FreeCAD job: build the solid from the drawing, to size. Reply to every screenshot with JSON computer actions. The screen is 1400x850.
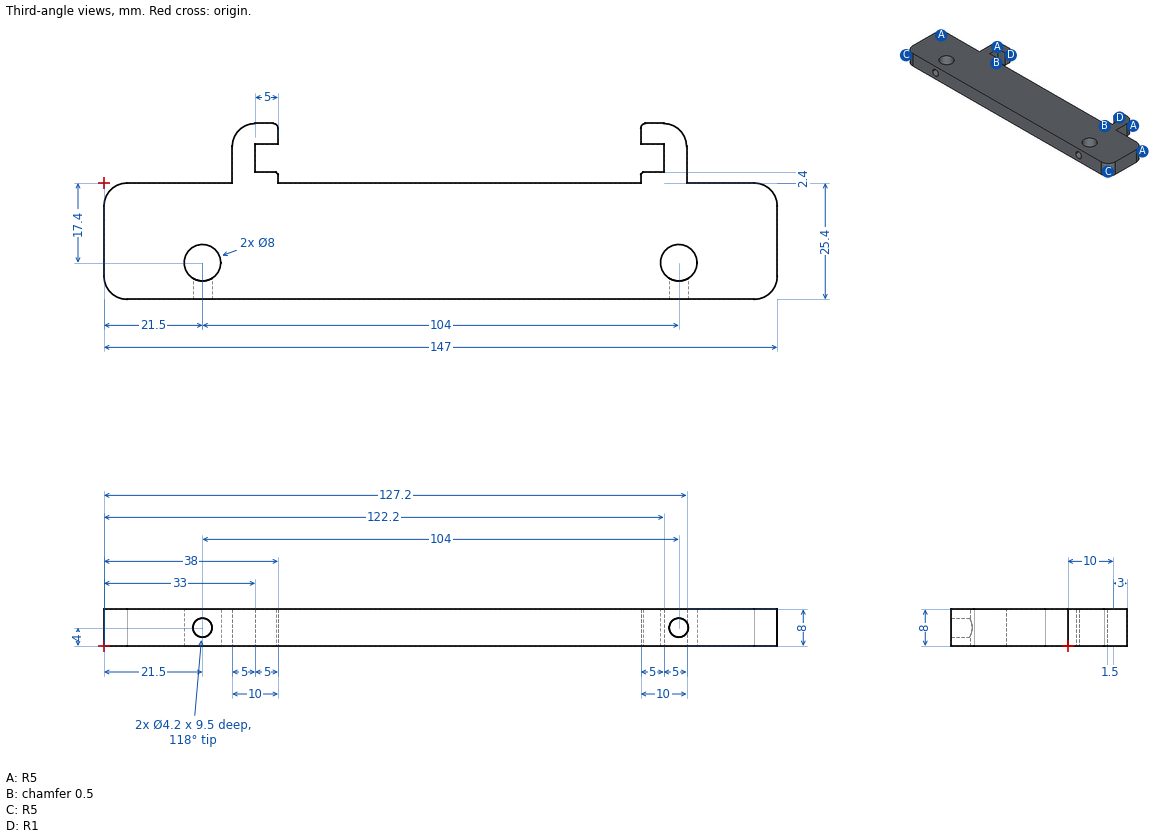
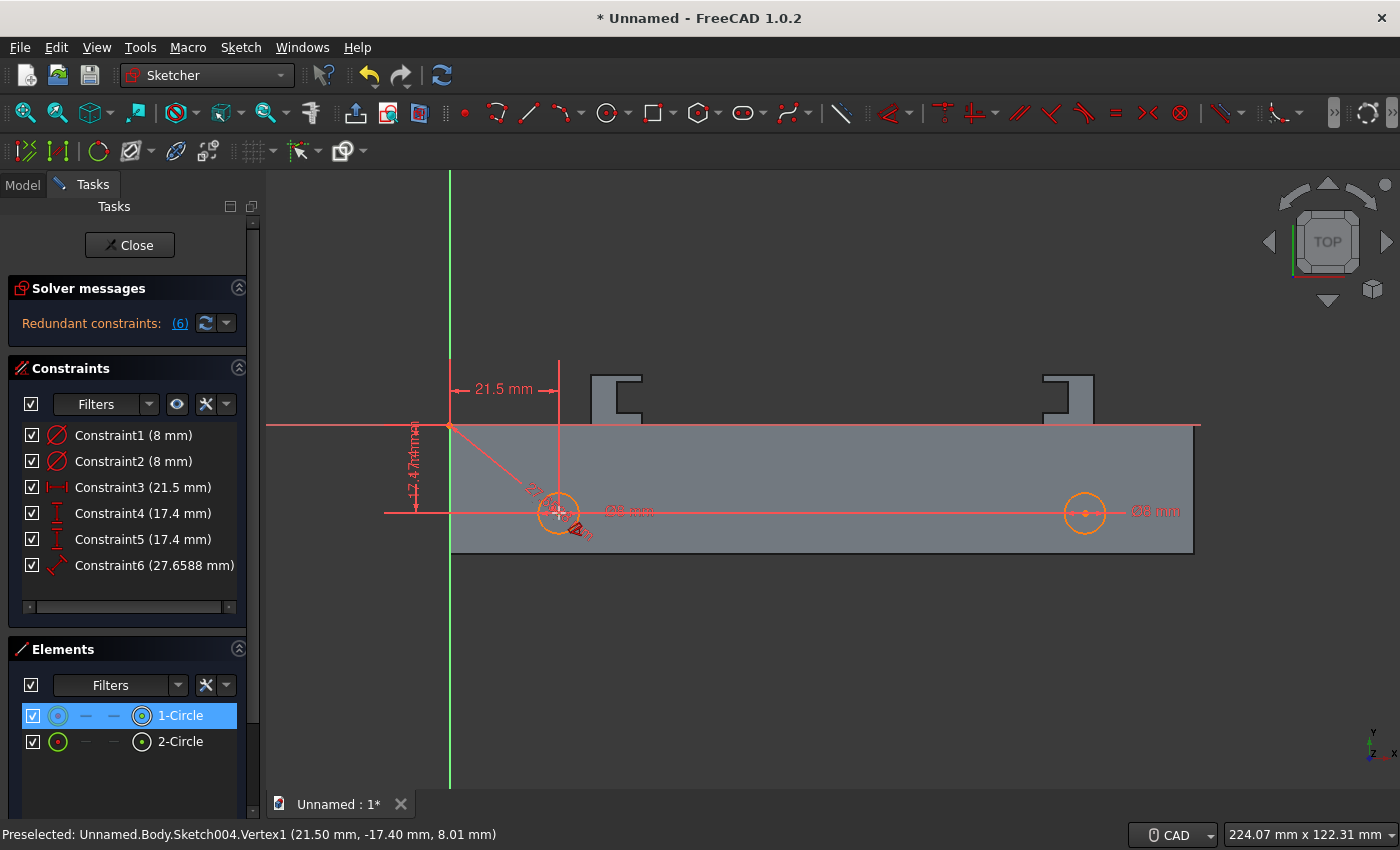
{"action": "left_click", "coordinate": [1085, 513]}
{"action": "left_click", "coordinate": [822, 547]}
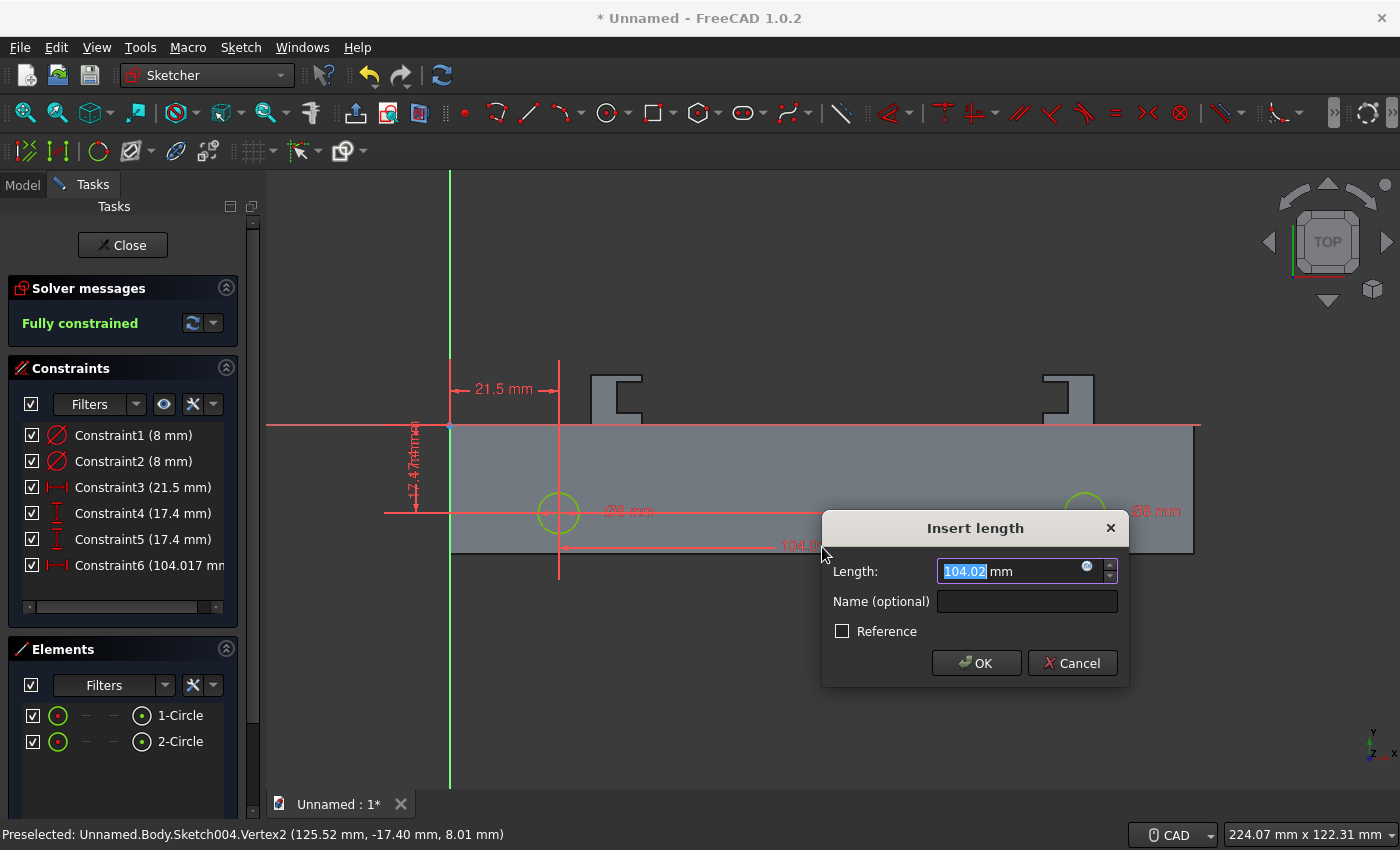
{"action": "type", "text": "104"}
{"action": "key", "text": "Return"}
{"action": "key", "text": "Escape"}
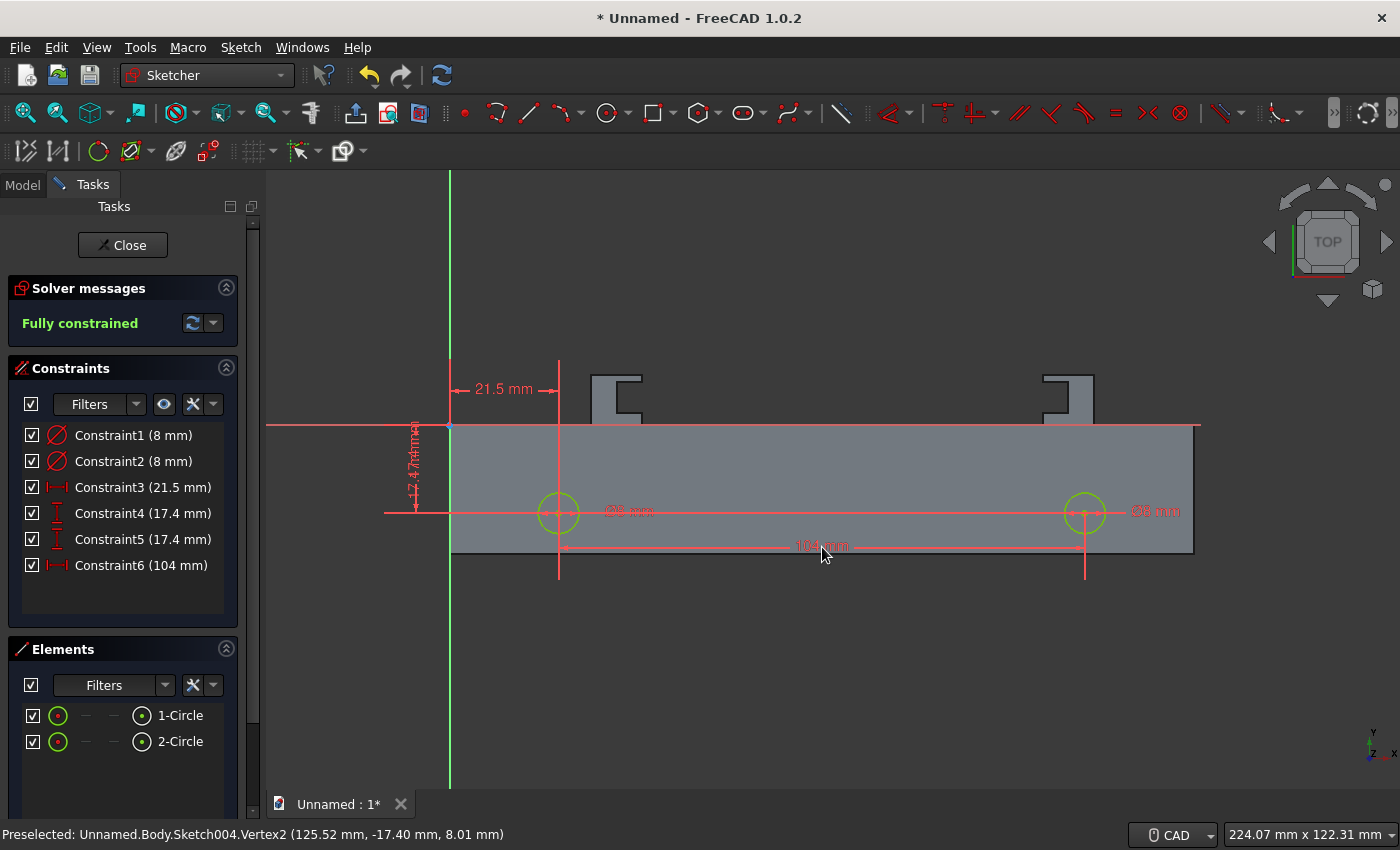
{"action": "left_click", "coordinate": [123, 245]}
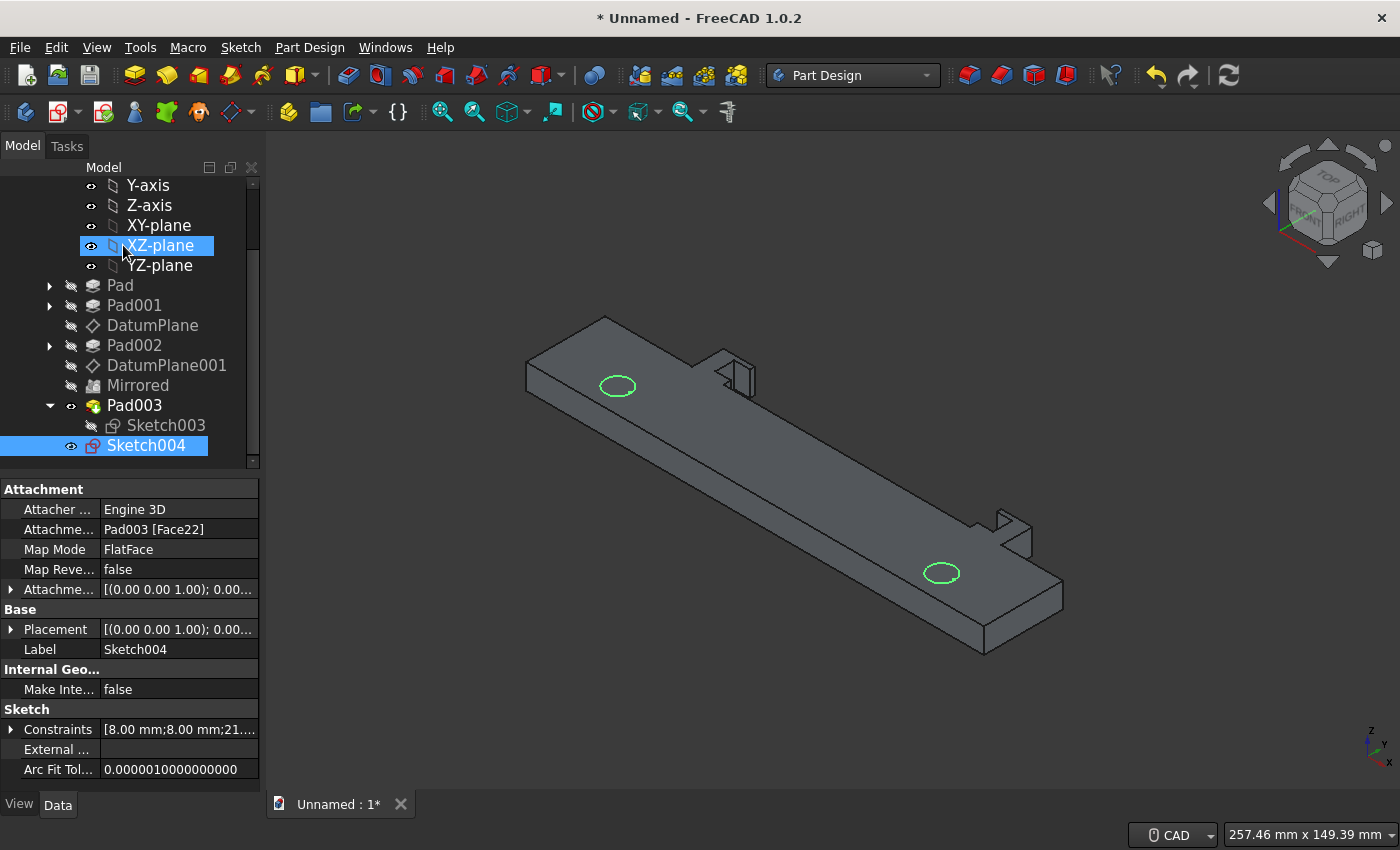
{"action": "left_click", "coordinate": [350, 76]}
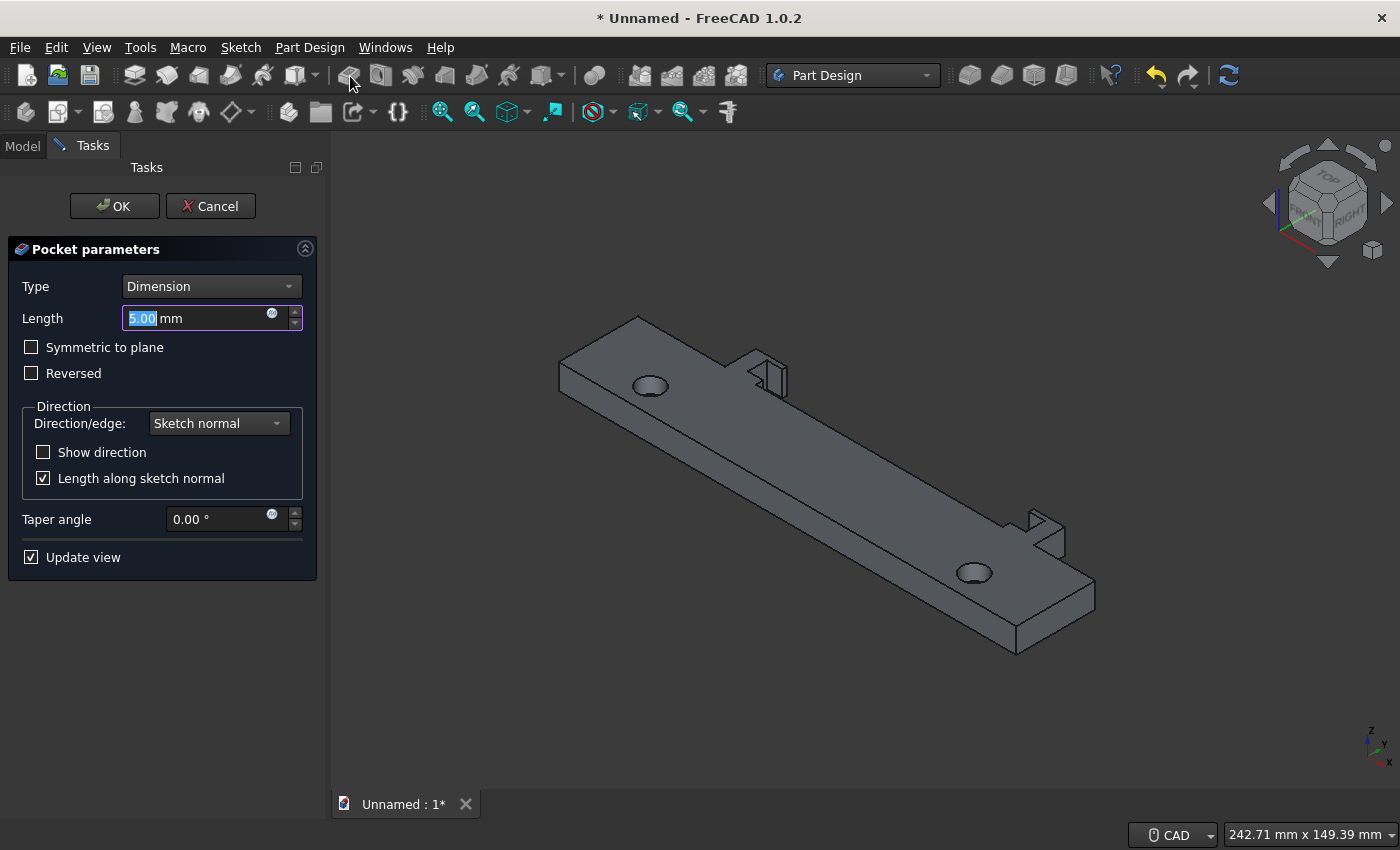
{"action": "left_click", "coordinate": [212, 286]}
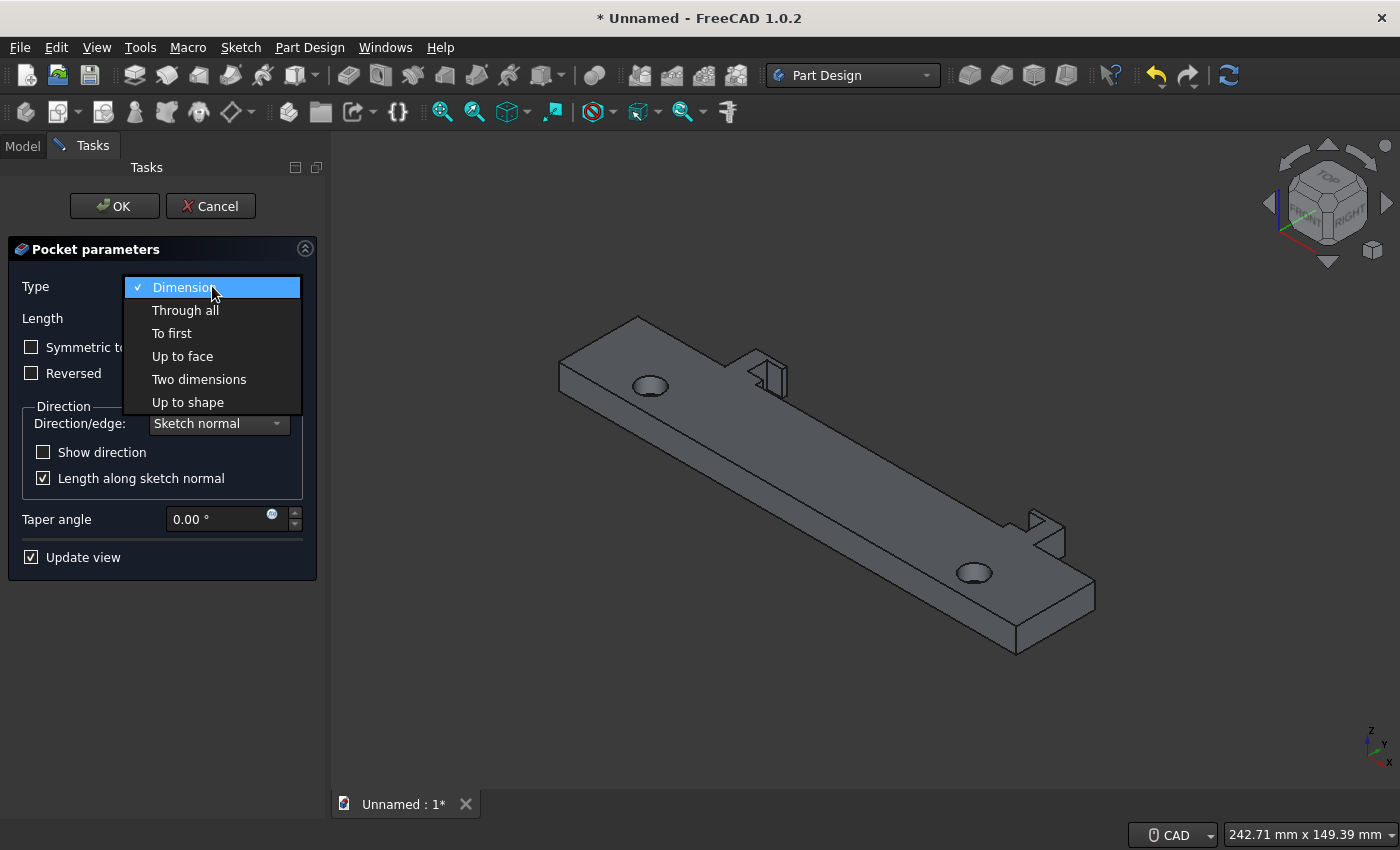
{"action": "left_click", "coordinate": [212, 310]}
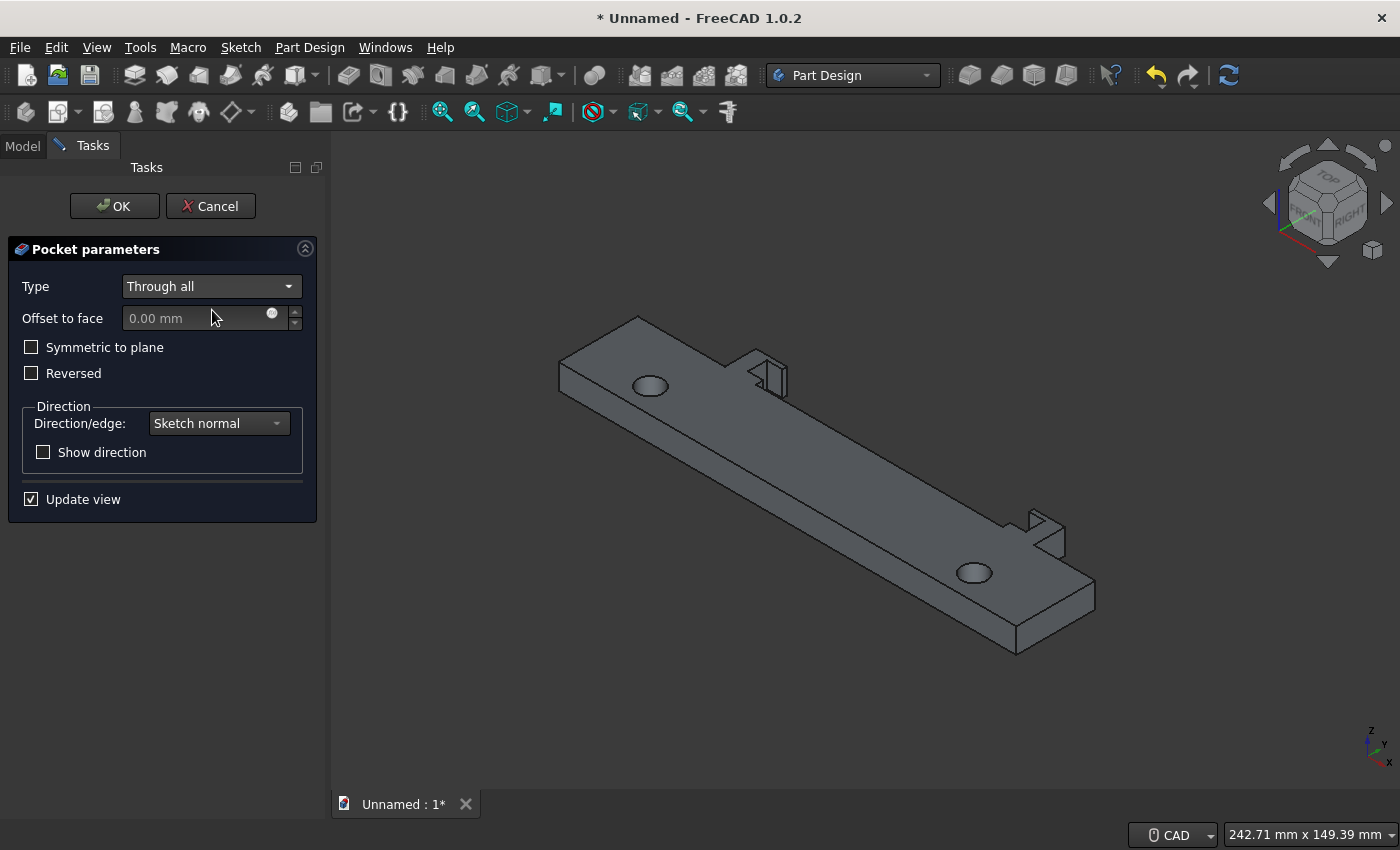
{"action": "left_click", "coordinate": [115, 206]}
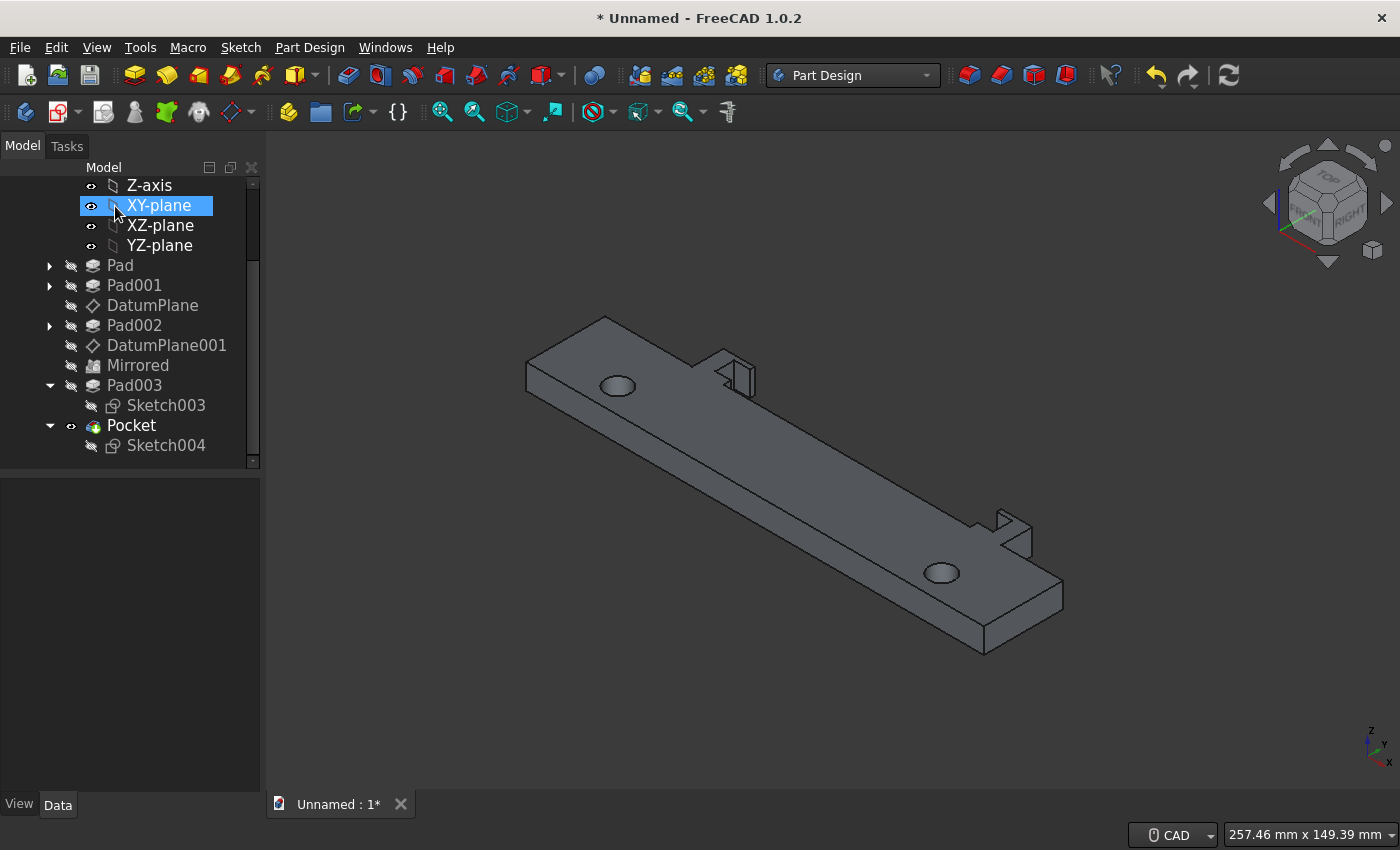
{"action": "key", "text": "4"}